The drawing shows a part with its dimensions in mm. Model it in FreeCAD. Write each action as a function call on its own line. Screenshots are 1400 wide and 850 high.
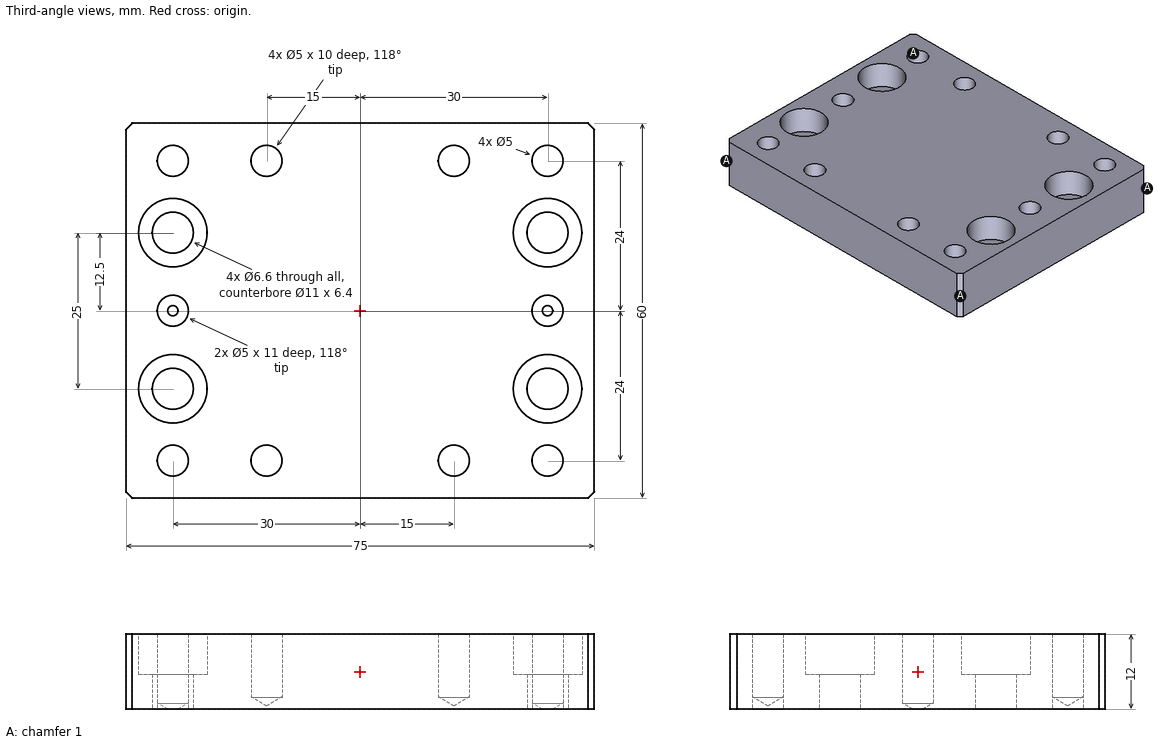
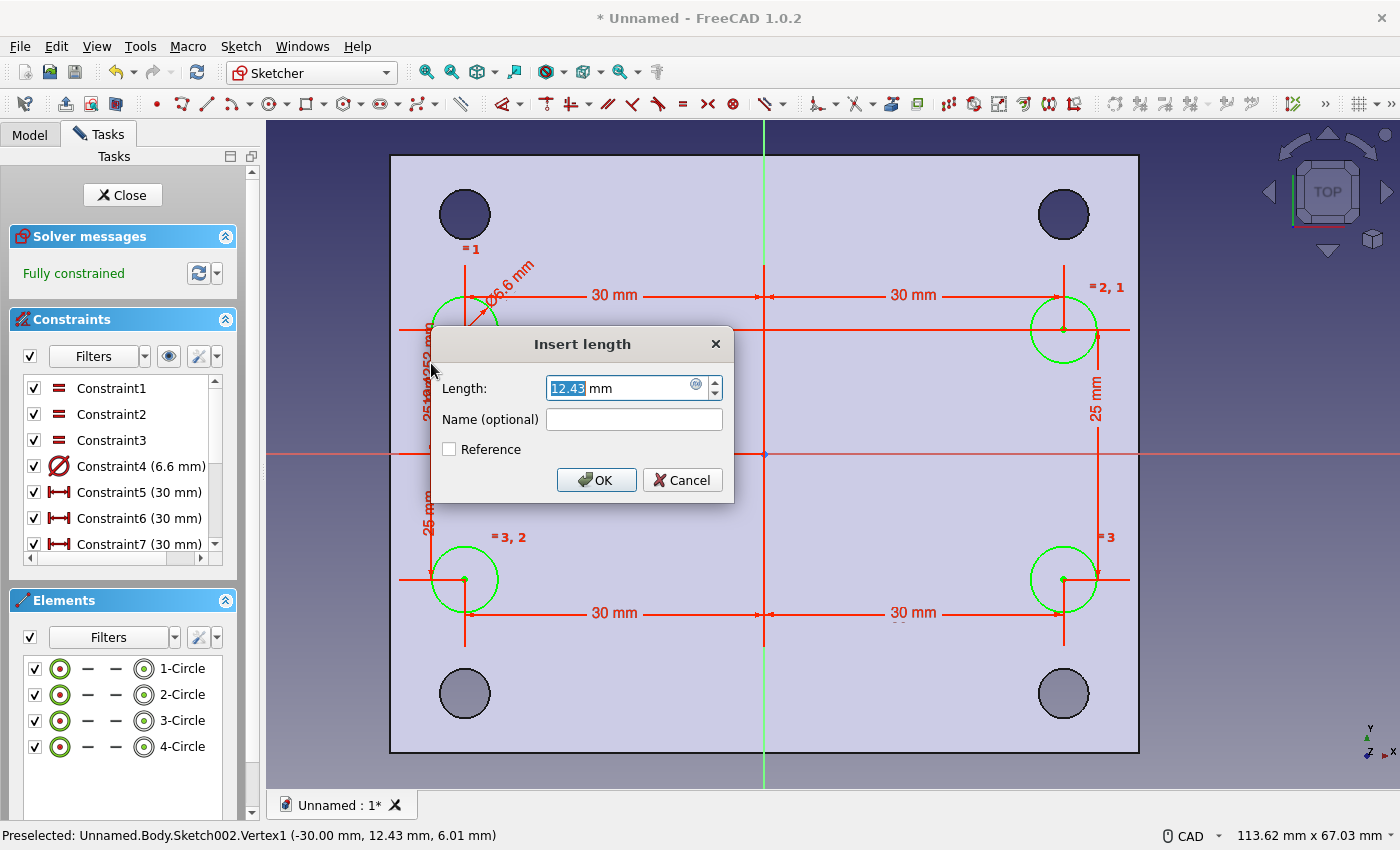
text(12.5)
key(Return)
key(Escape)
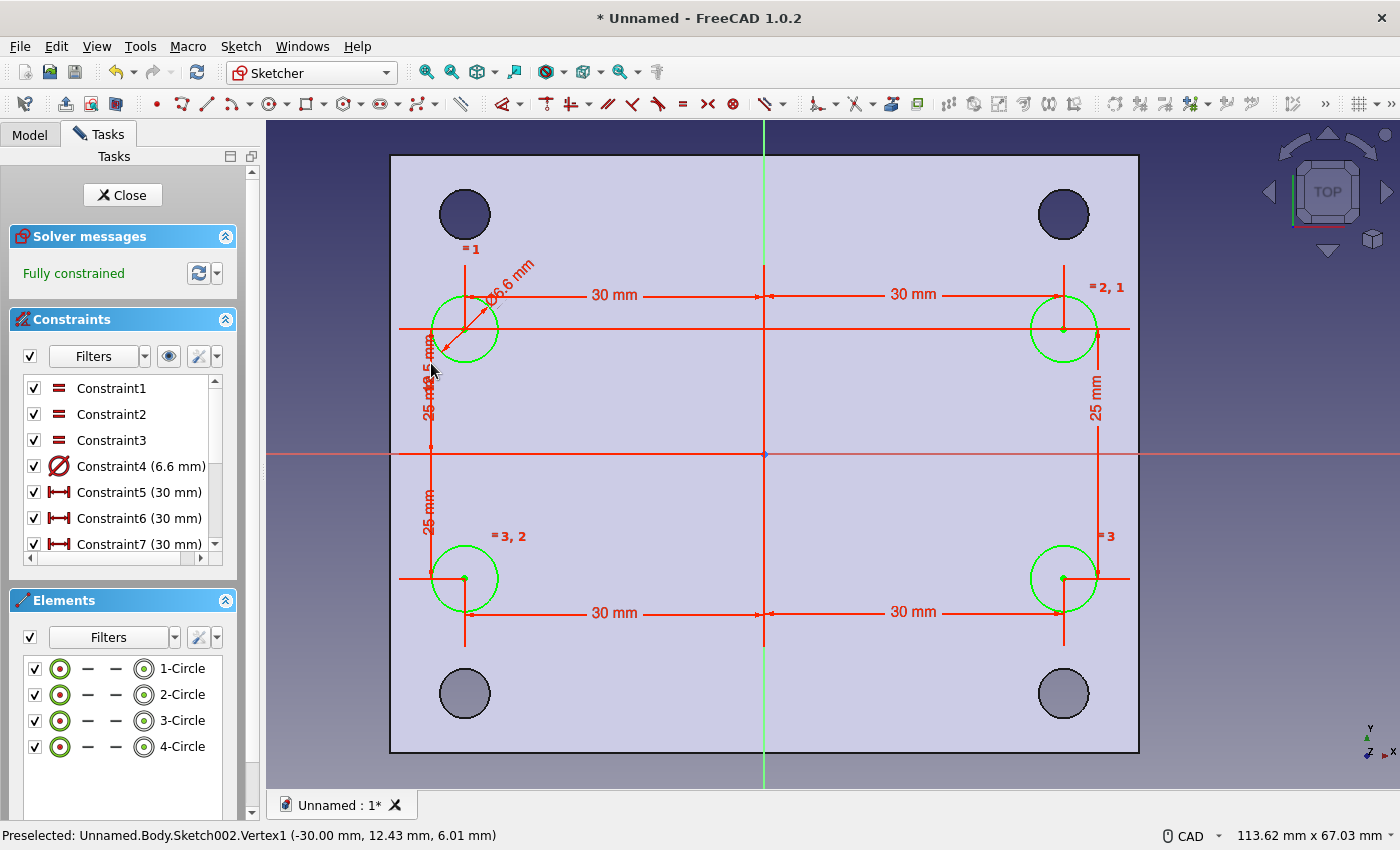
click(123, 195)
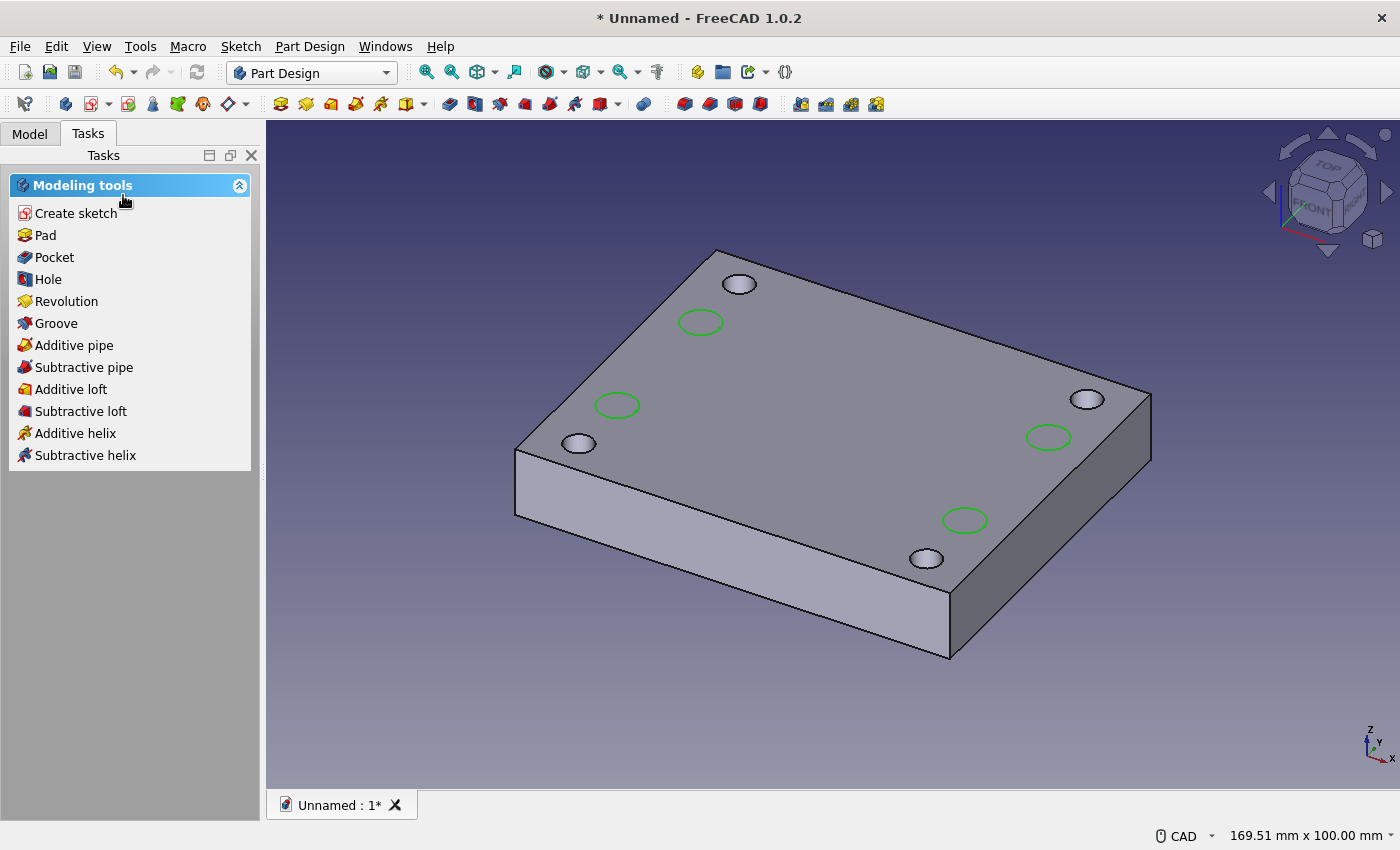
click(475, 104)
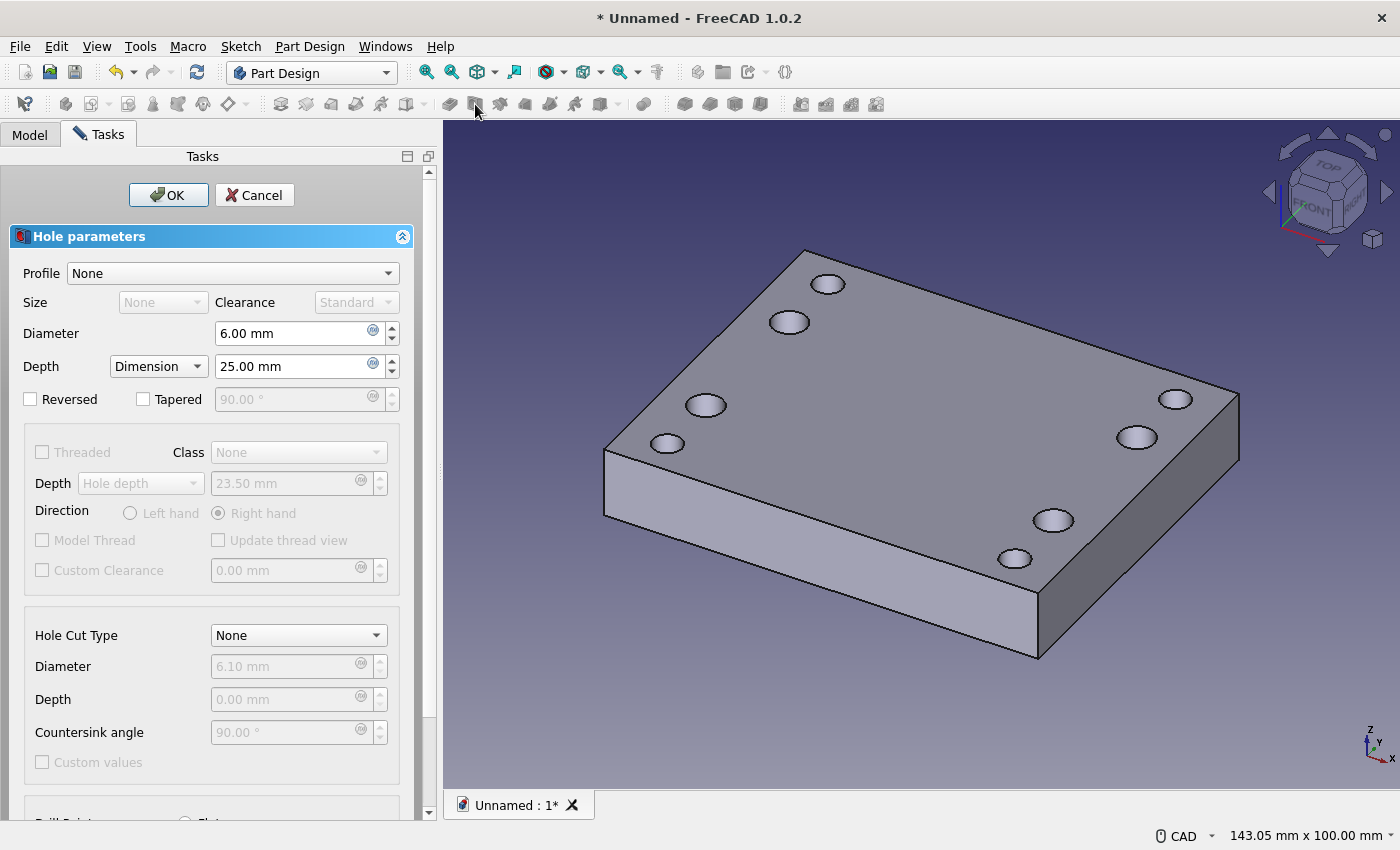
triple_click(300, 334)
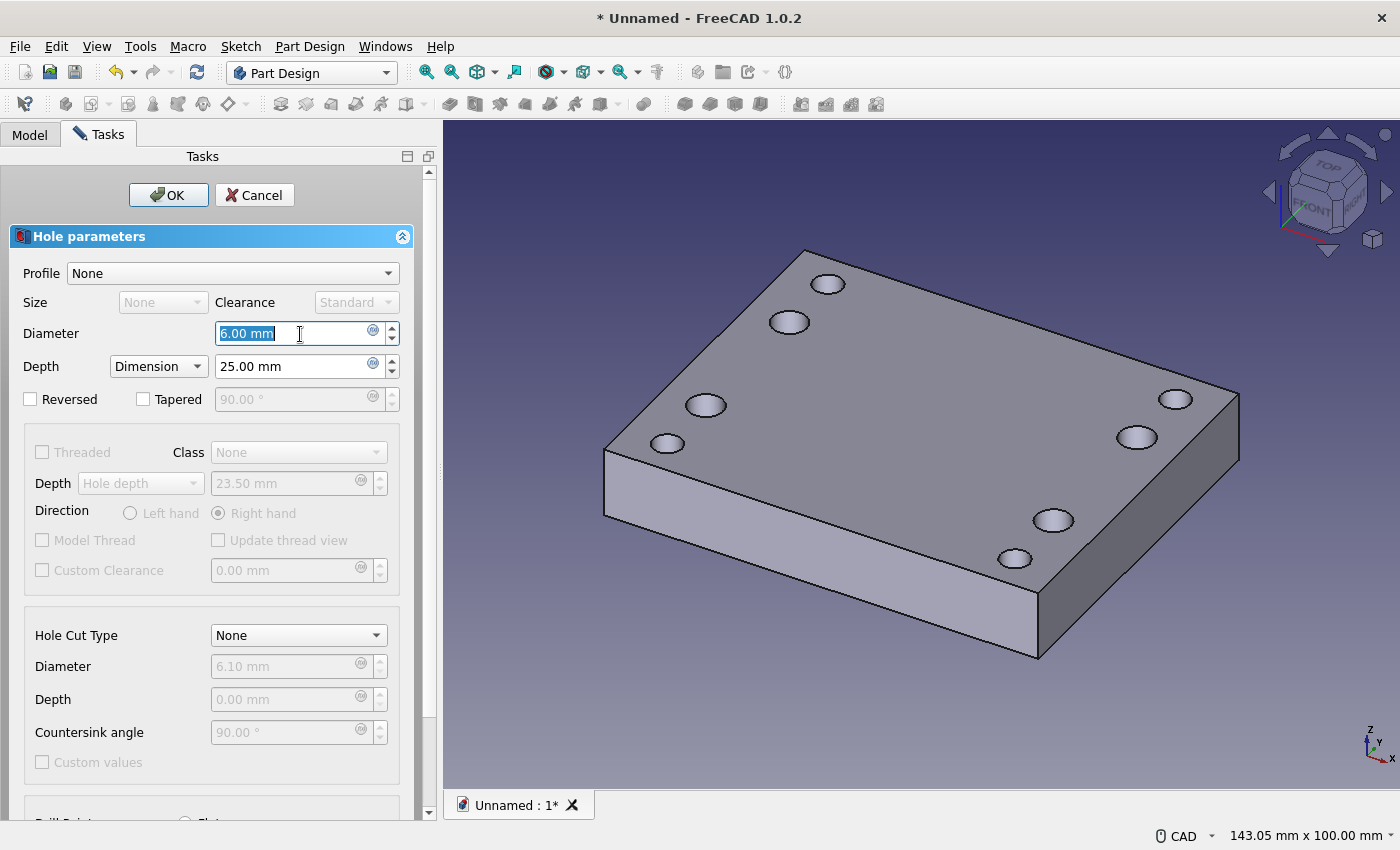
text(6.6)
key(Tab)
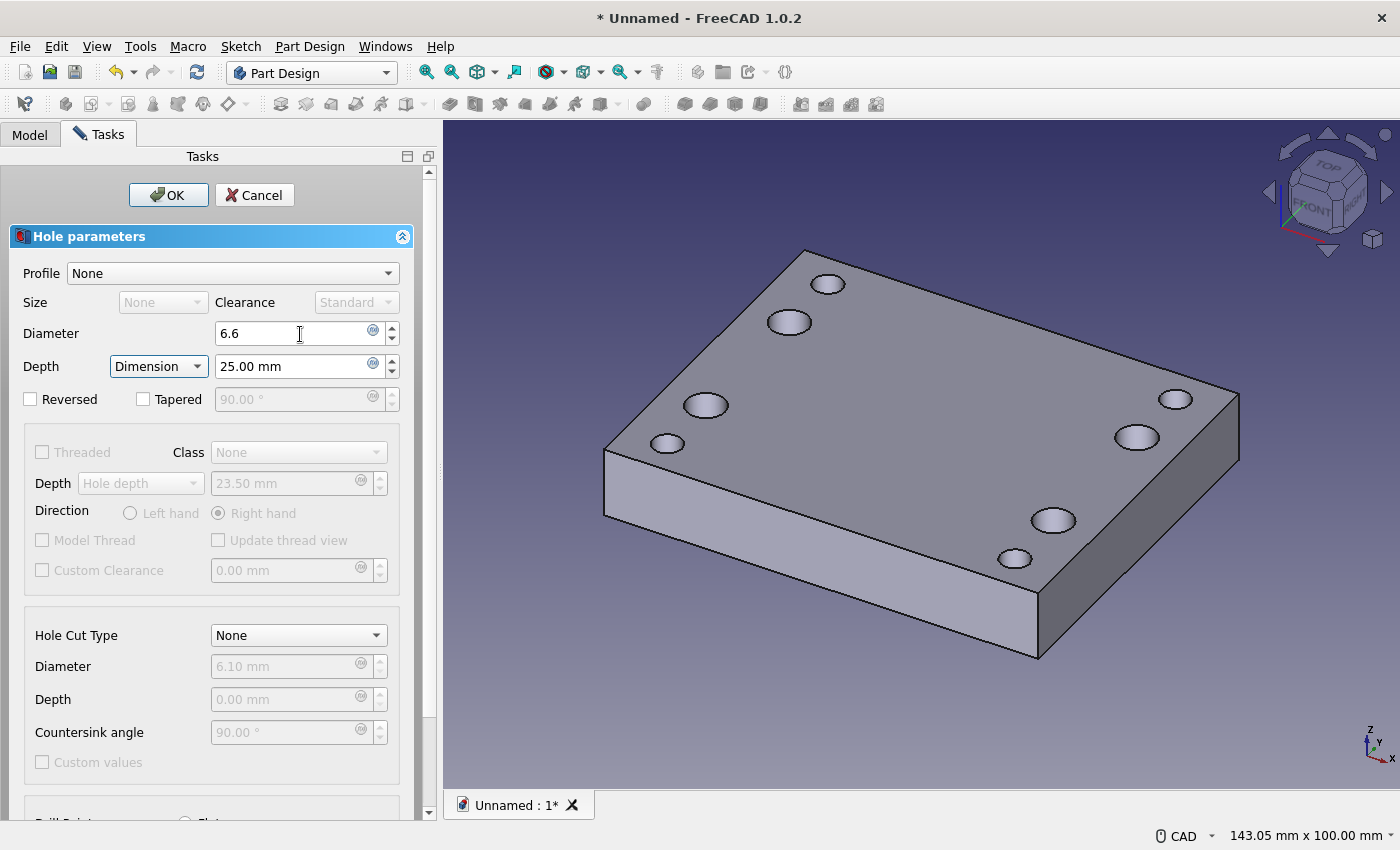
click(160, 366)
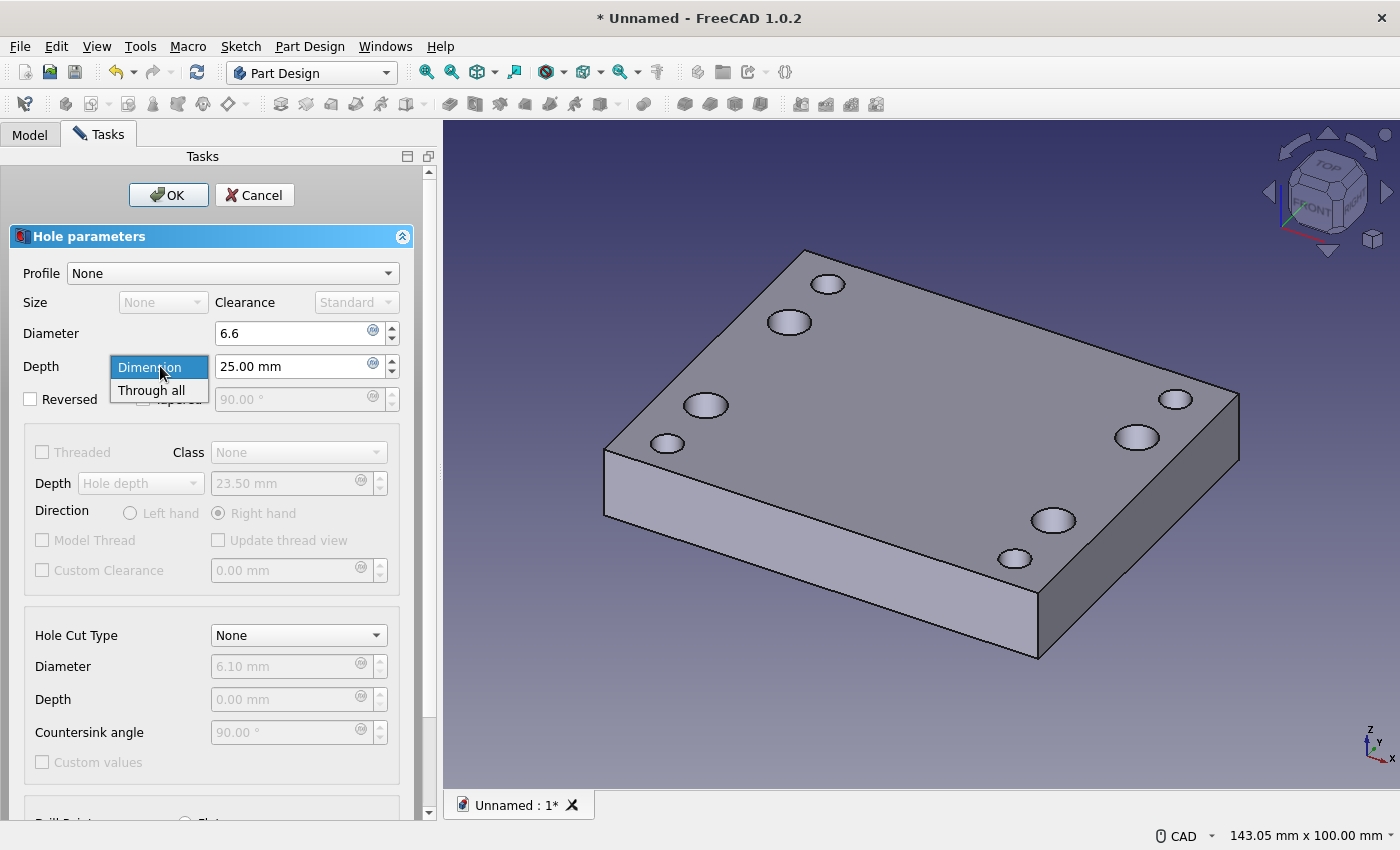
click(158, 390)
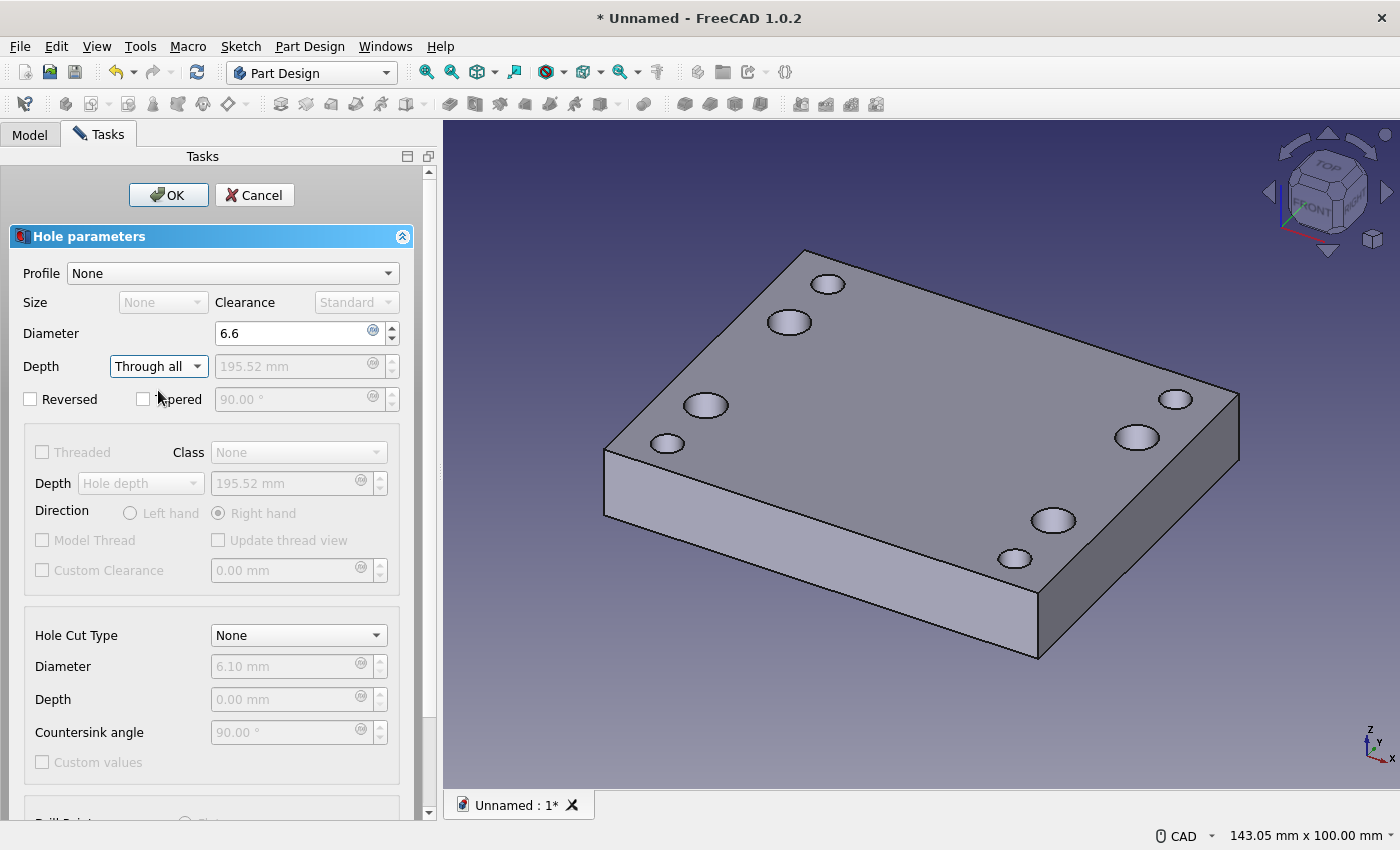
click(300, 636)